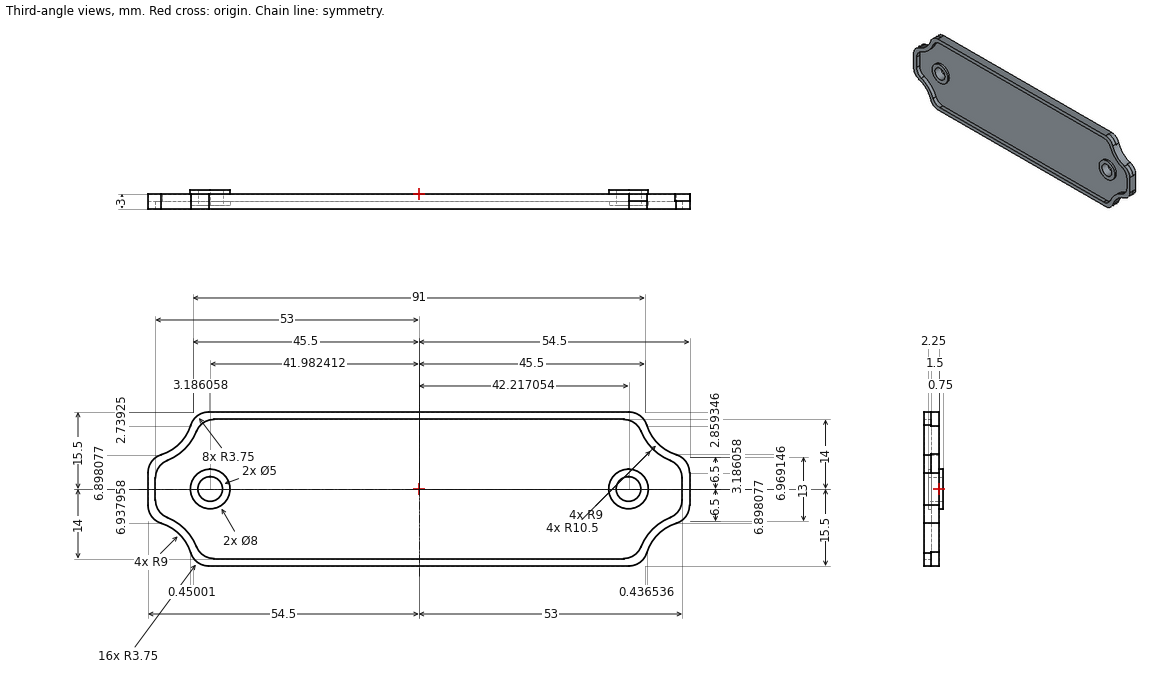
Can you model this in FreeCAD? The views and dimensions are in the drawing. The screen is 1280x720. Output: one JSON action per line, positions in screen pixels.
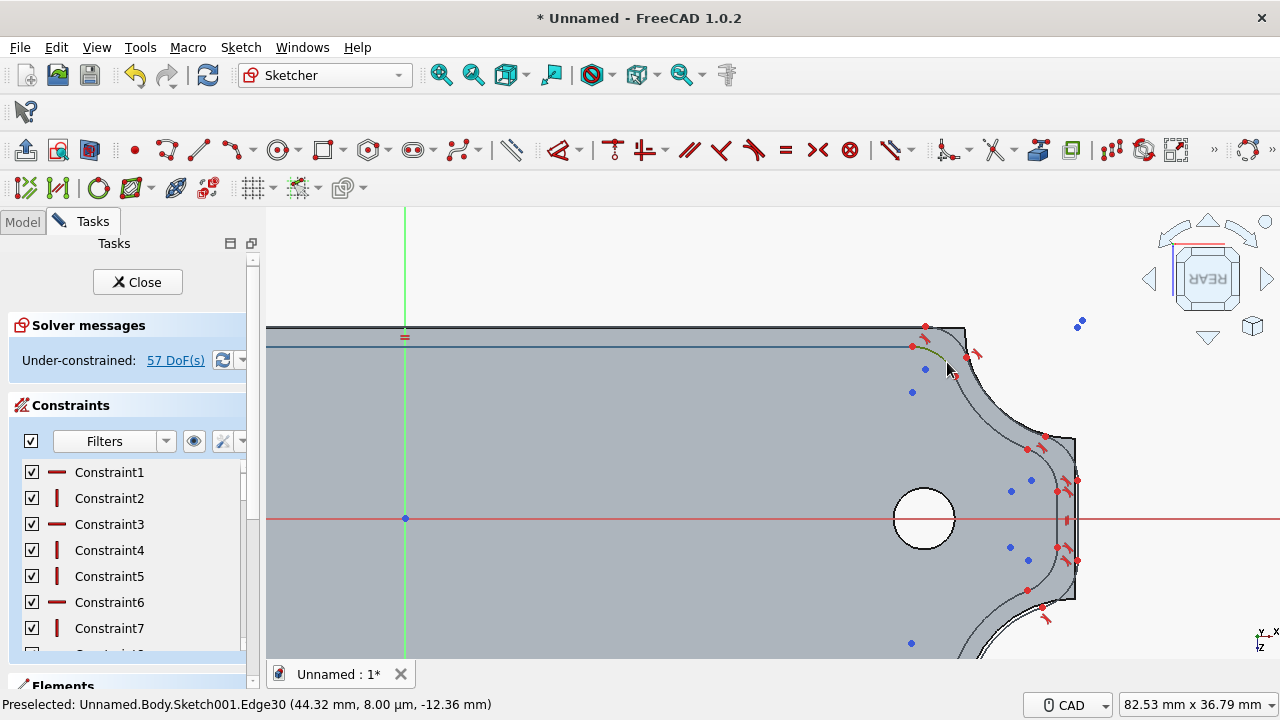
{"action": "left_click", "coordinate": [754, 150]}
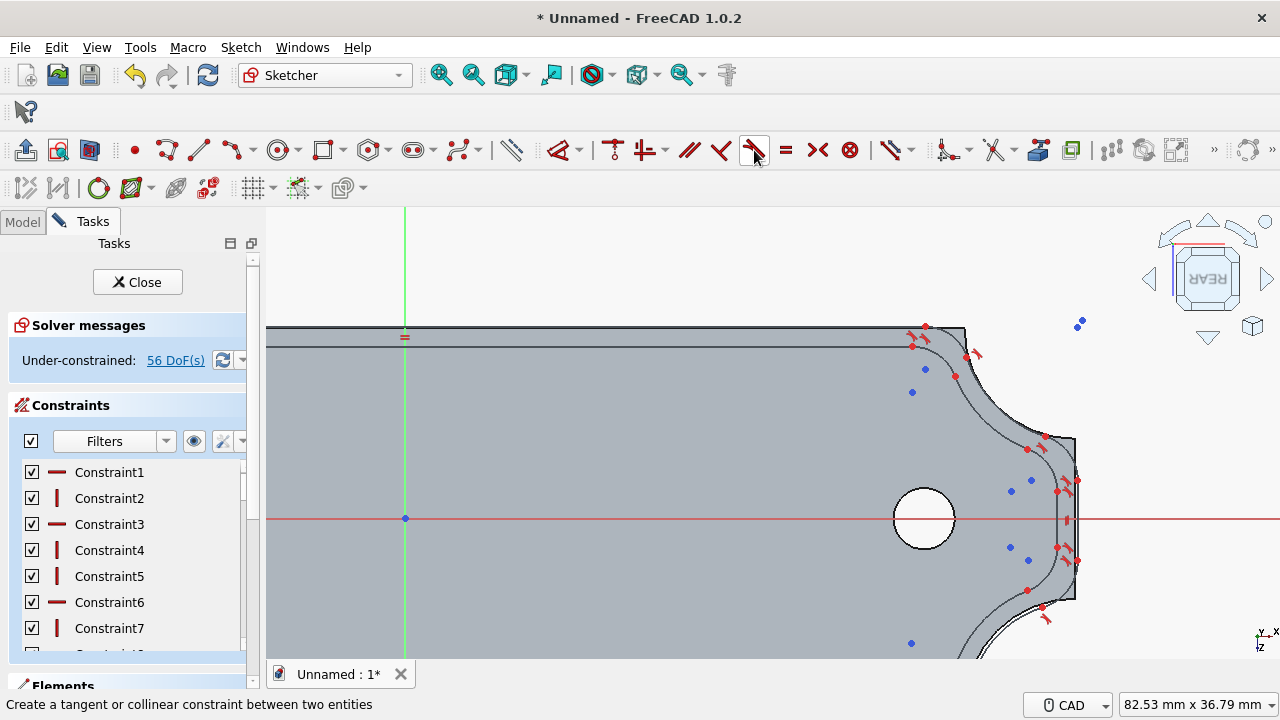
{"action": "left_click", "coordinate": [1042, 582]}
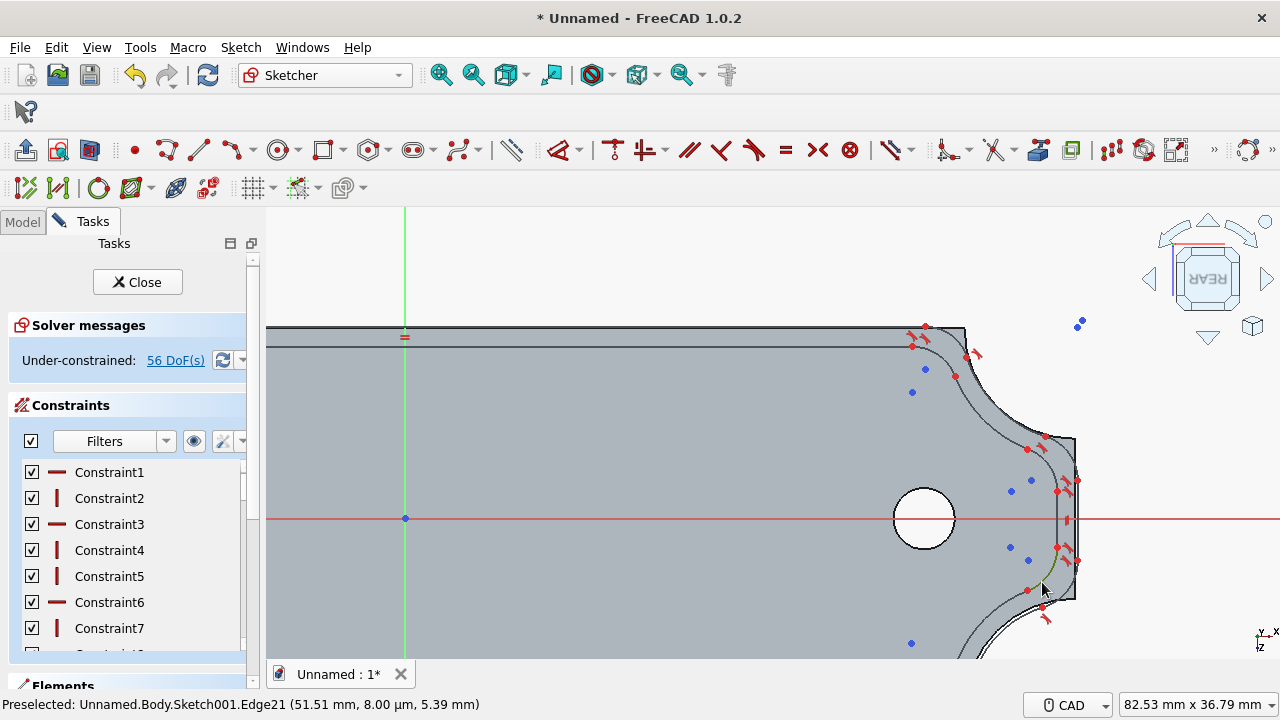
{"action": "left_click", "coordinate": [1000, 606]}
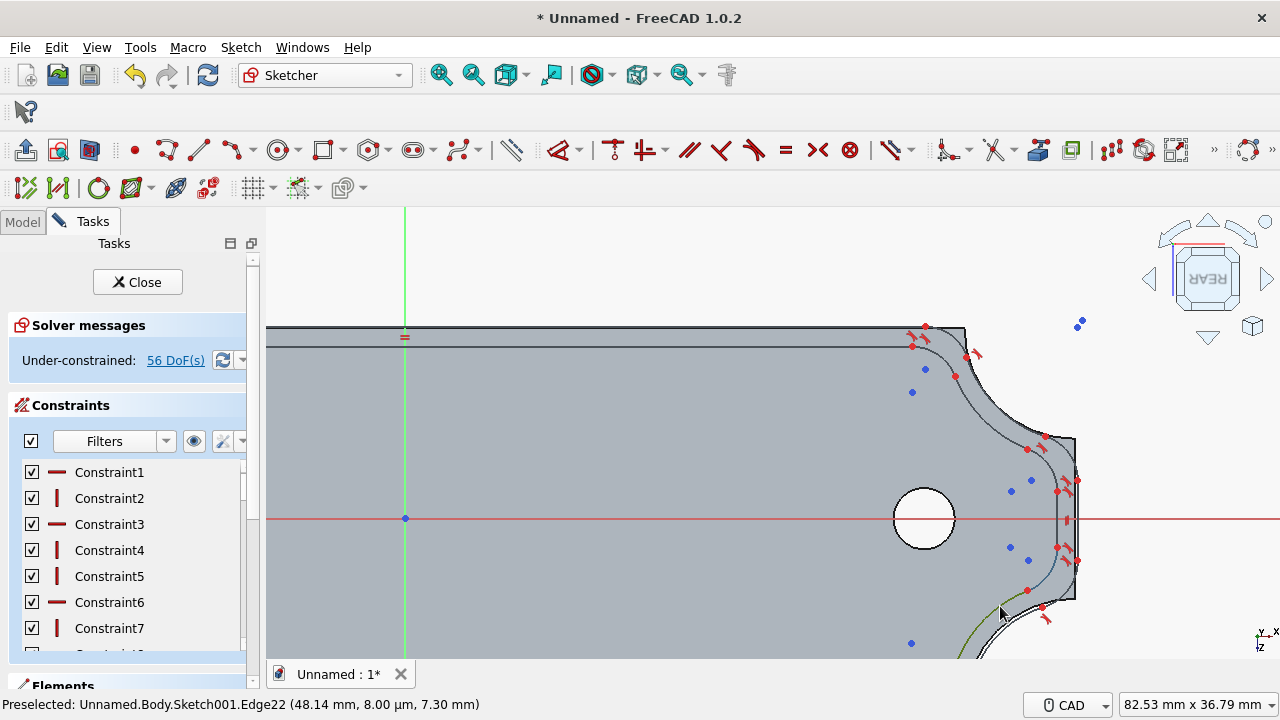
{"action": "left_click", "coordinate": [754, 150]}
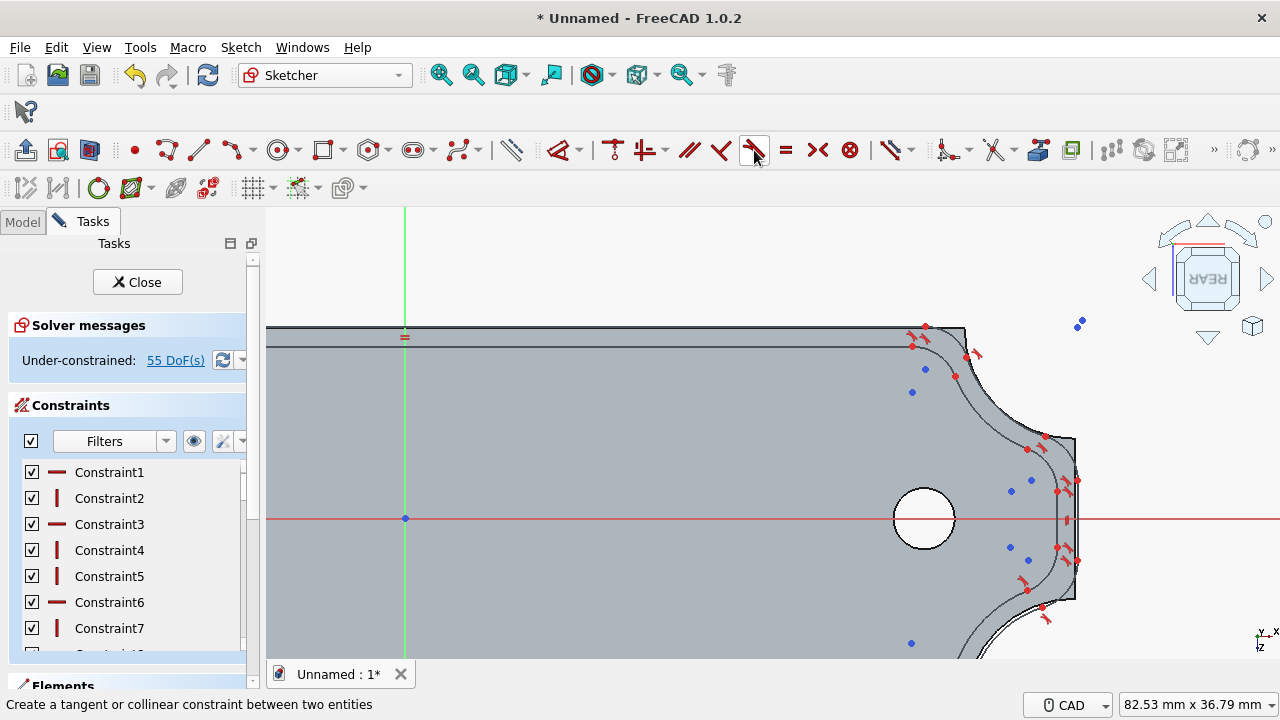
{"action": "left_click", "coordinate": [1000, 606]}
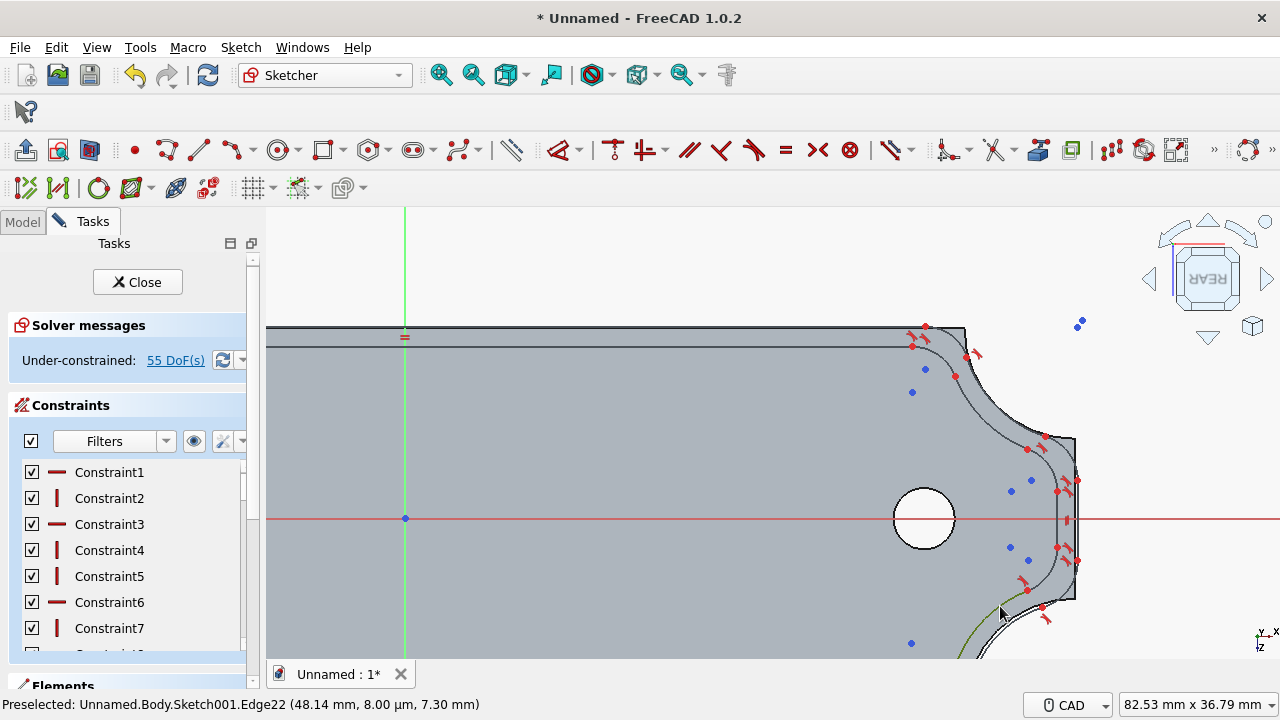
{"action": "scroll", "coordinate": [949, 363], "scroll_direction": "down", "scroll_amount": 4}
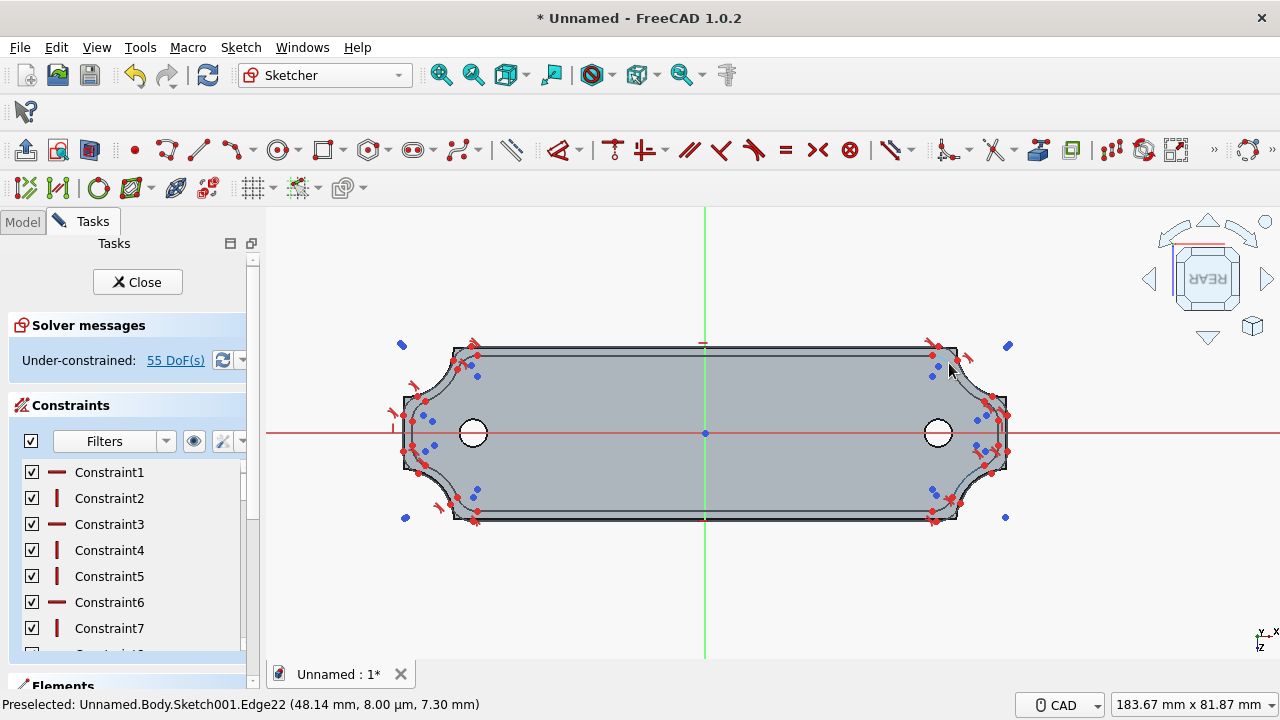
{"action": "scroll", "coordinate": [940, 510], "scroll_direction": "up", "scroll_amount": 3}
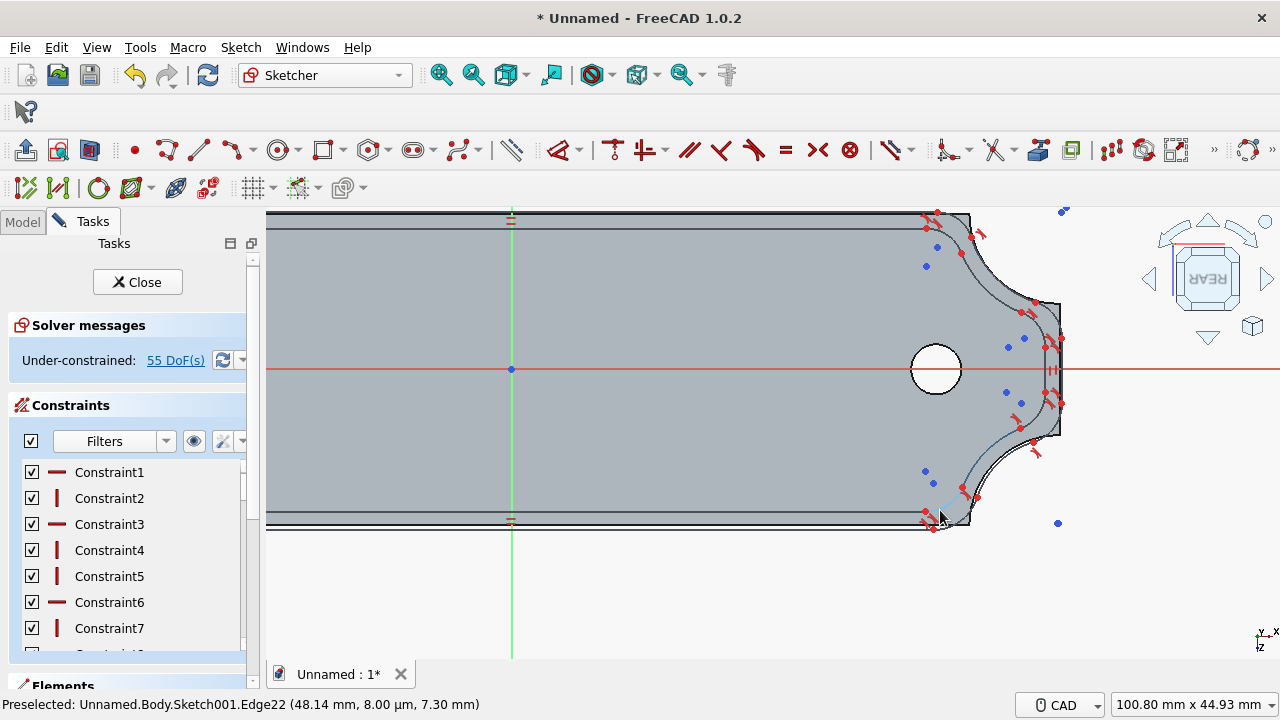
{"action": "left_click", "coordinate": [939, 509]}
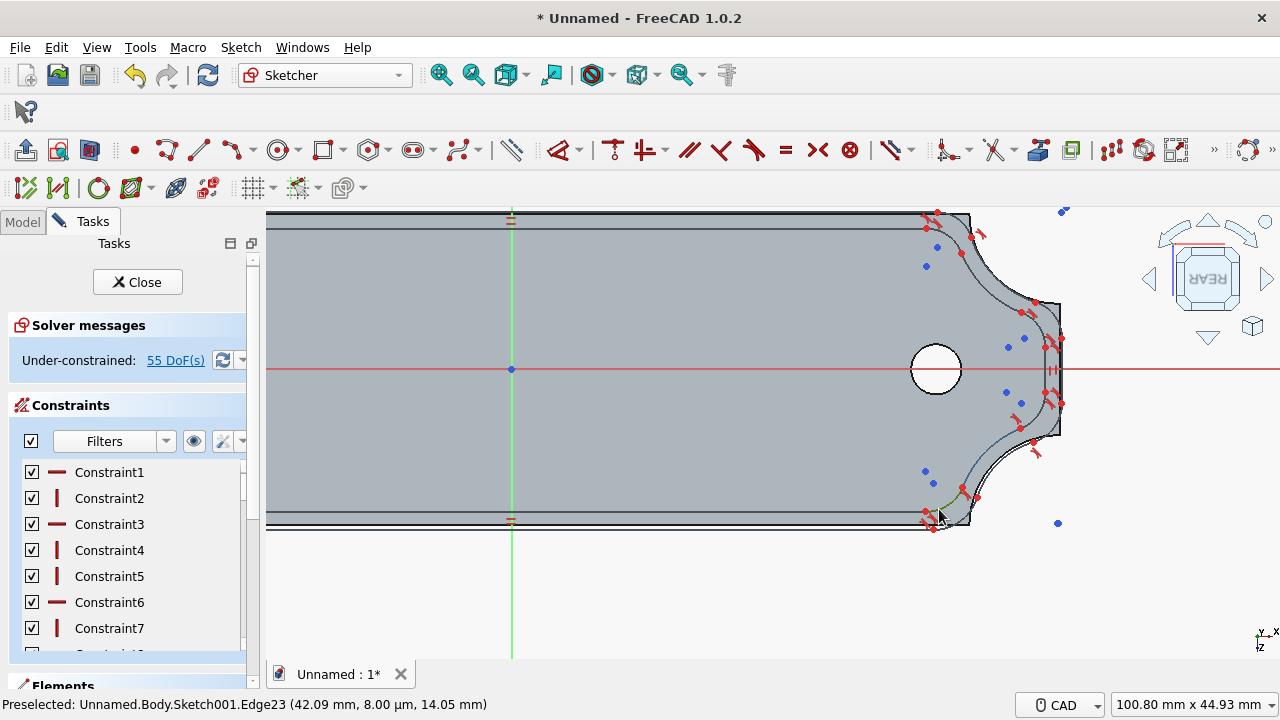
{"action": "left_click", "coordinate": [754, 150]}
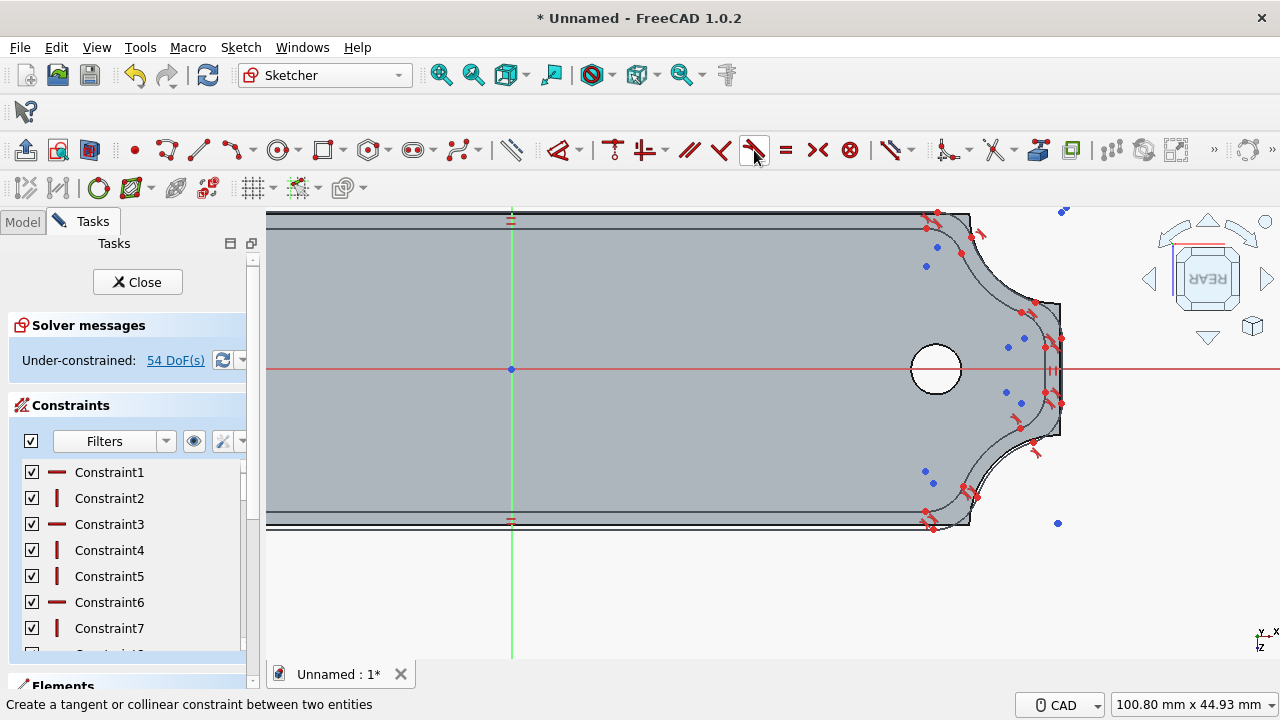
{"action": "scroll", "coordinate": [939, 510], "scroll_direction": "down", "scroll_amount": 3}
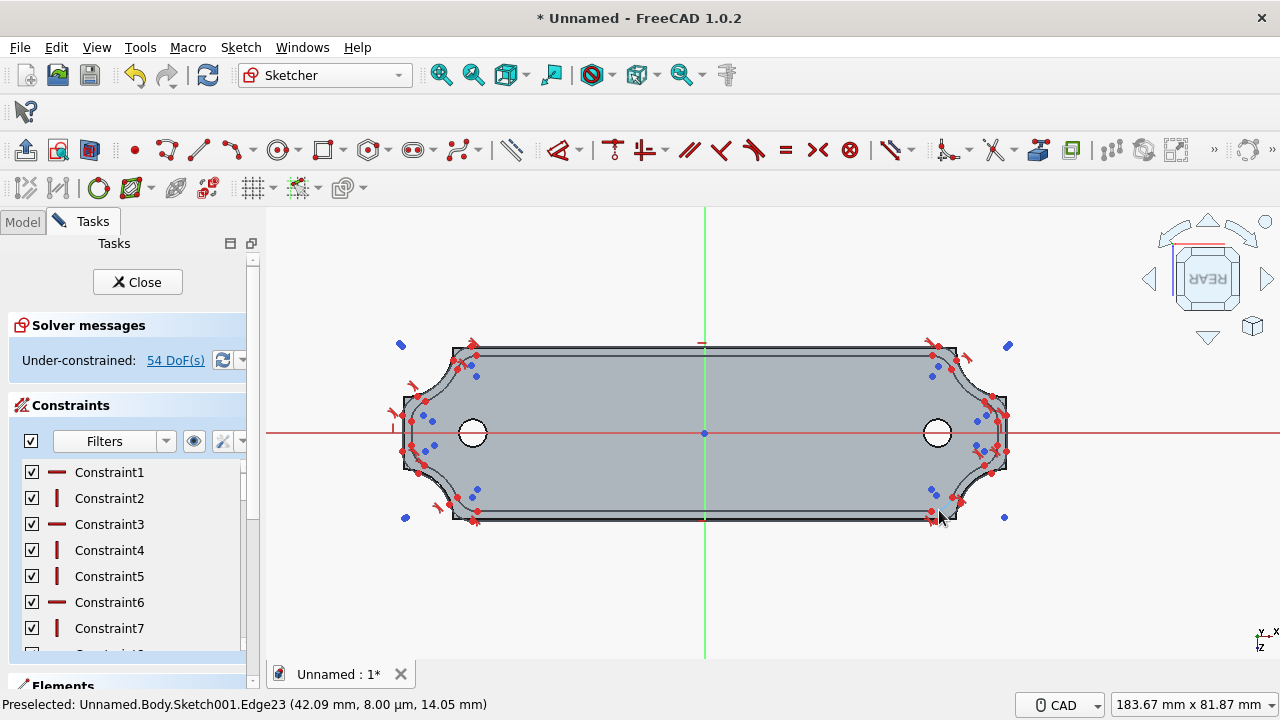
{"action": "scroll", "coordinate": [461, 504], "scroll_direction": "up", "scroll_amount": 3}